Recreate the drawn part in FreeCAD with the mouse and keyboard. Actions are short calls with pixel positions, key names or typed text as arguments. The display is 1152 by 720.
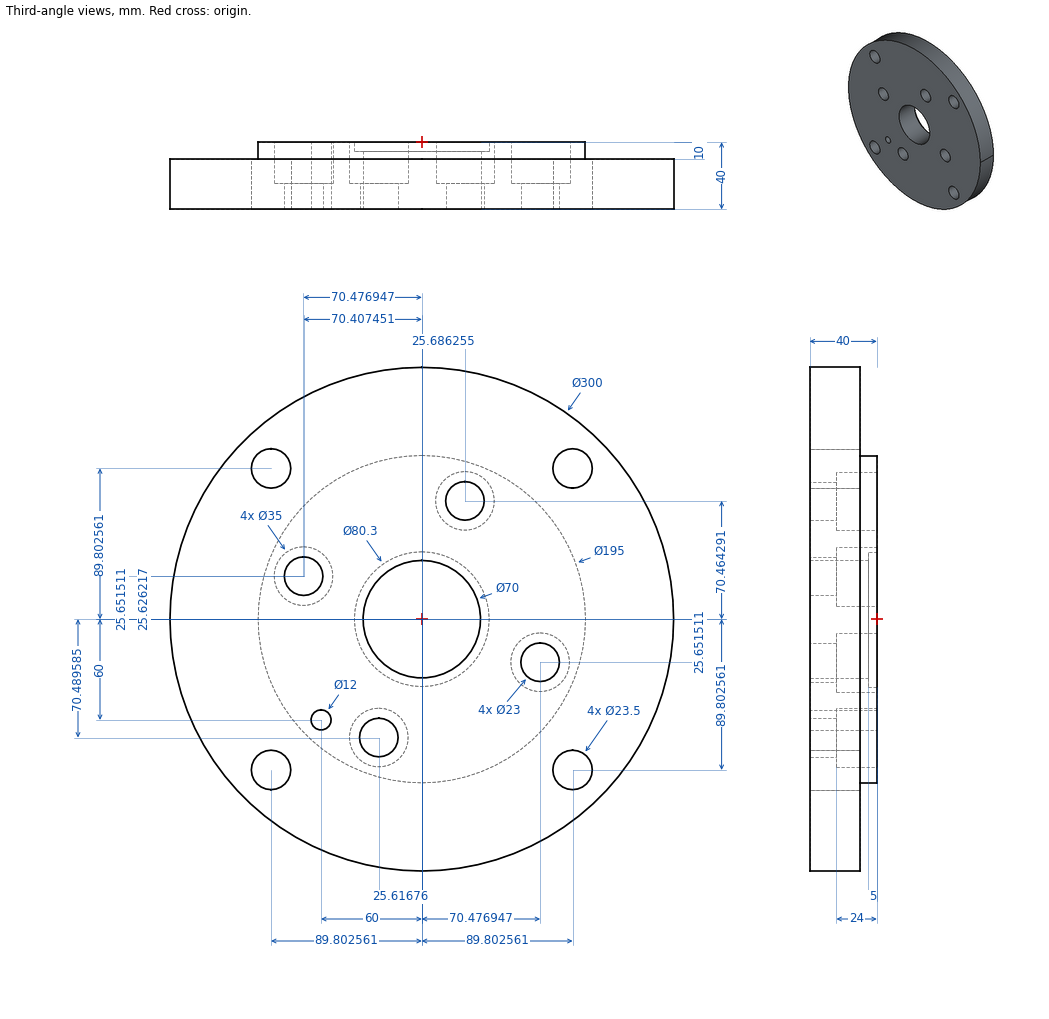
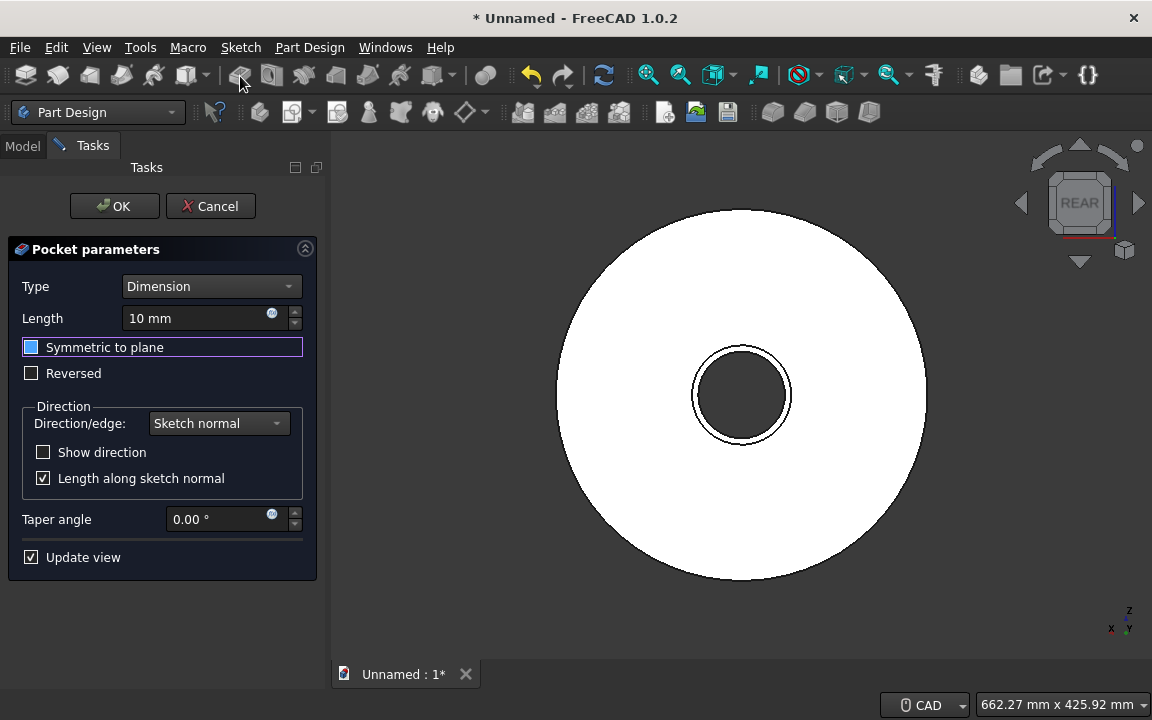
click(30, 373)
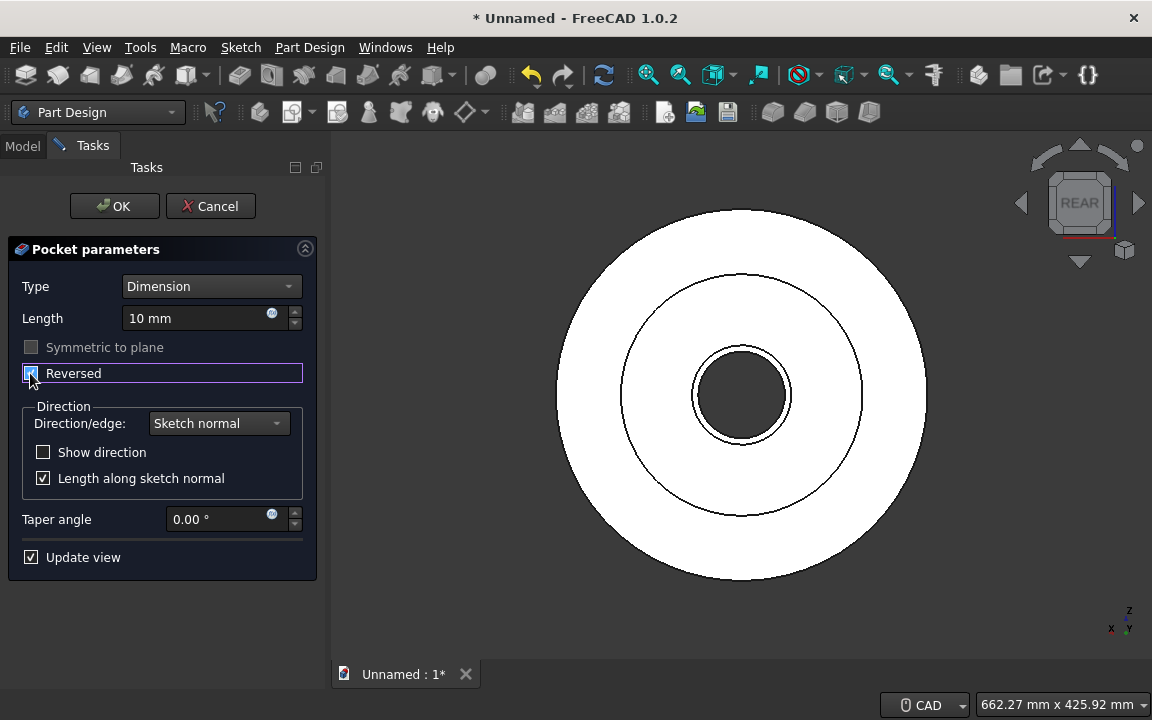
click(115, 206)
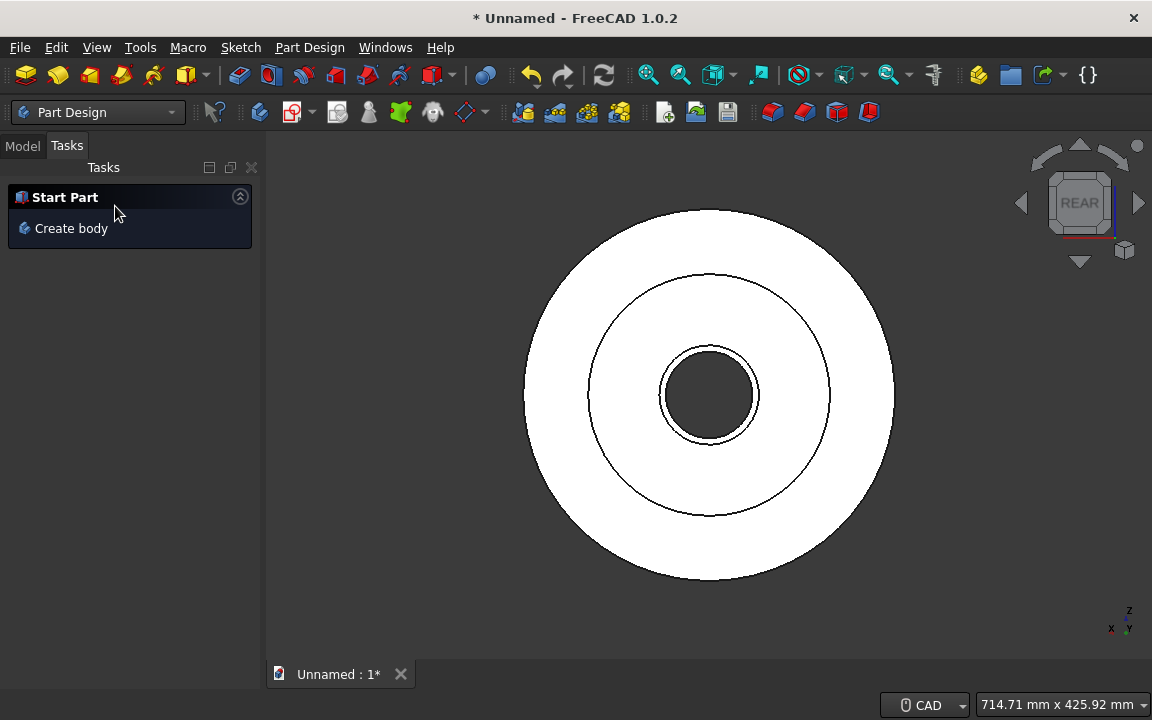
click(815, 288)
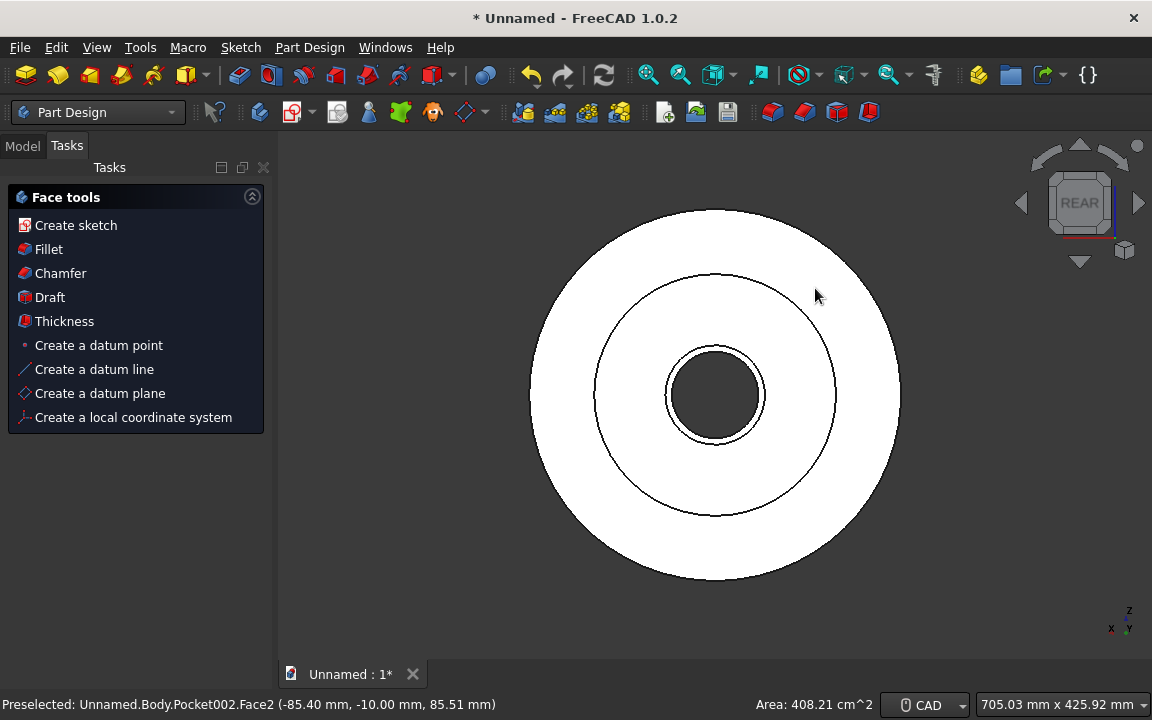
click(292, 112)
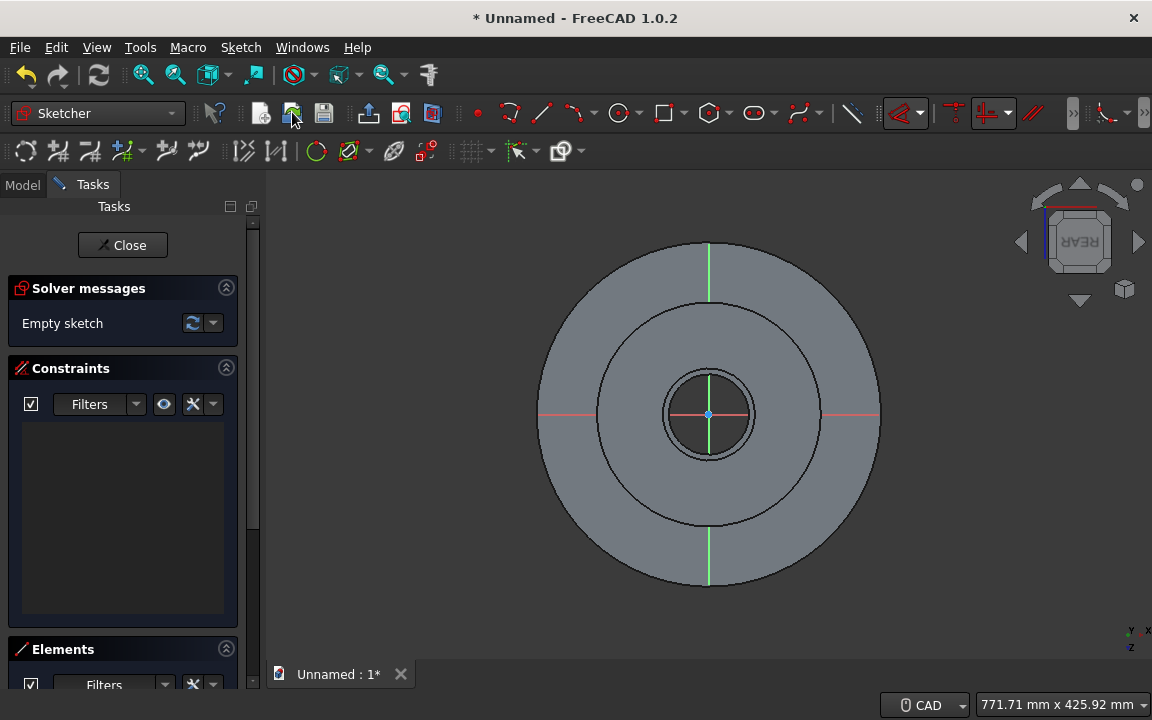
click(434, 114)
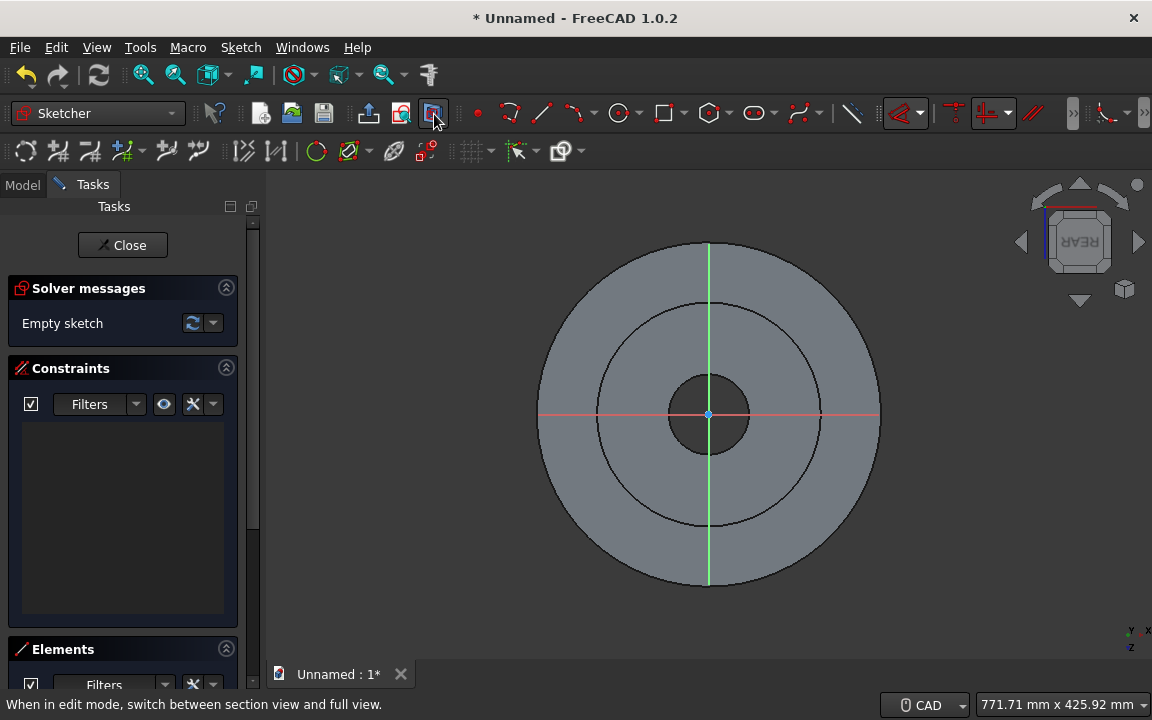
click(620, 114)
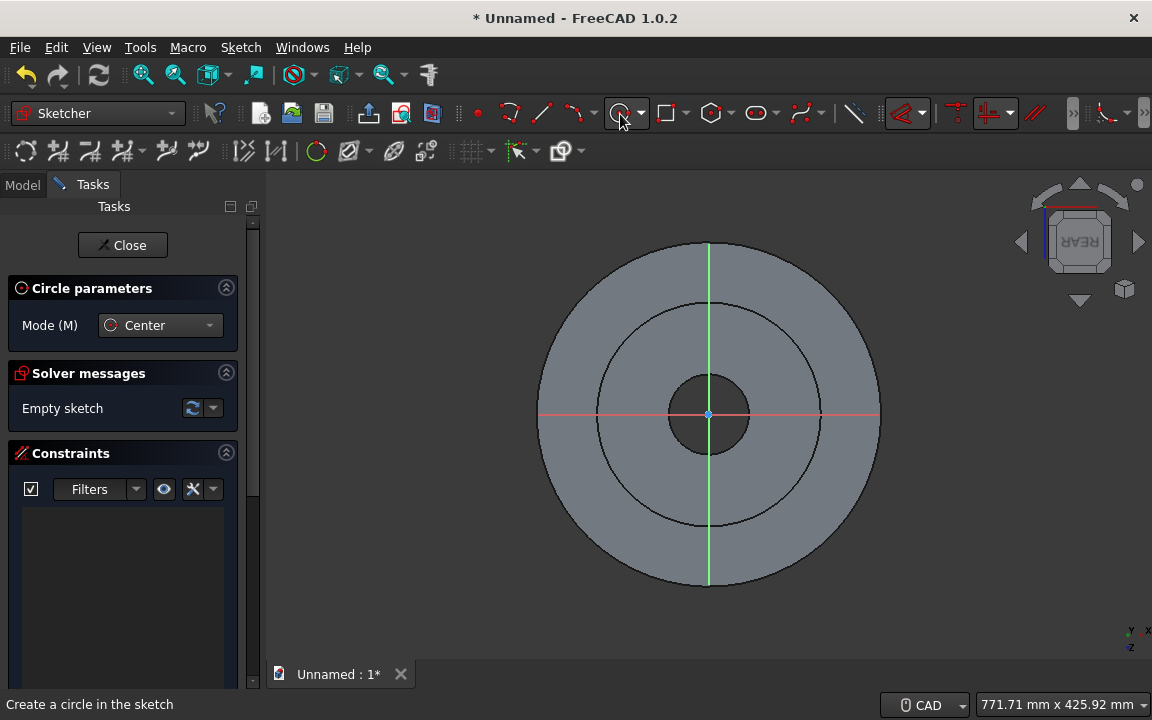
scroll(812, 311, up, 3)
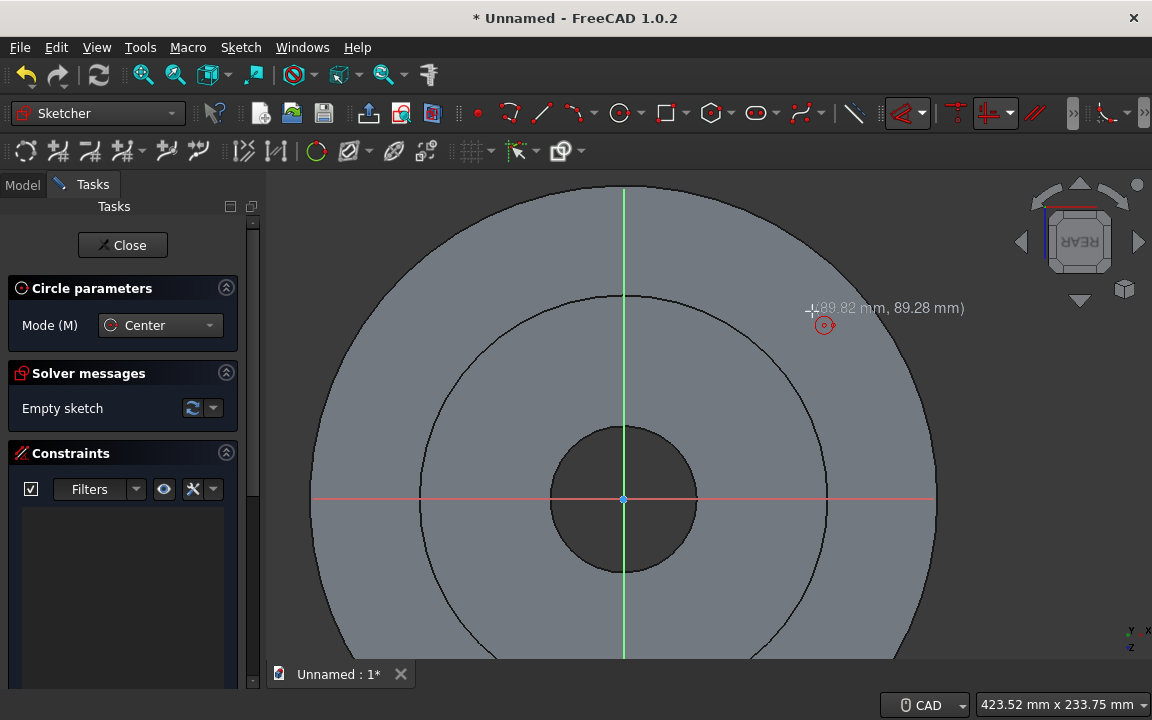
click(811, 311)
move(829, 294)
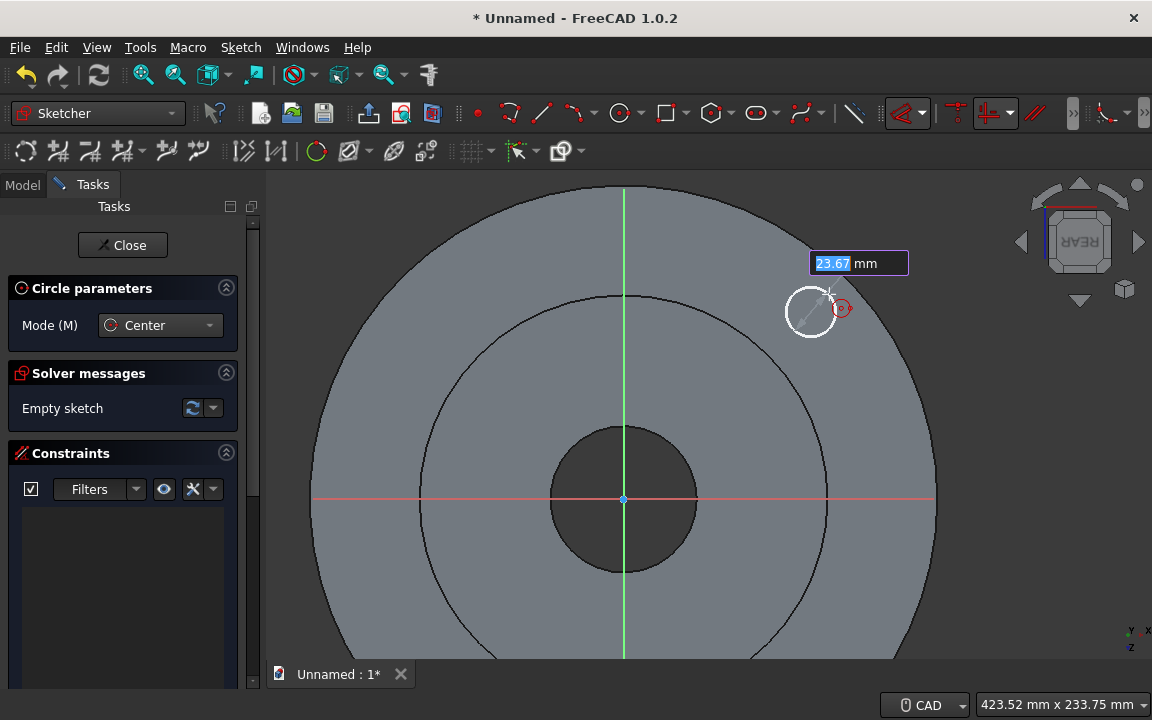
text(23.5)
key(Return)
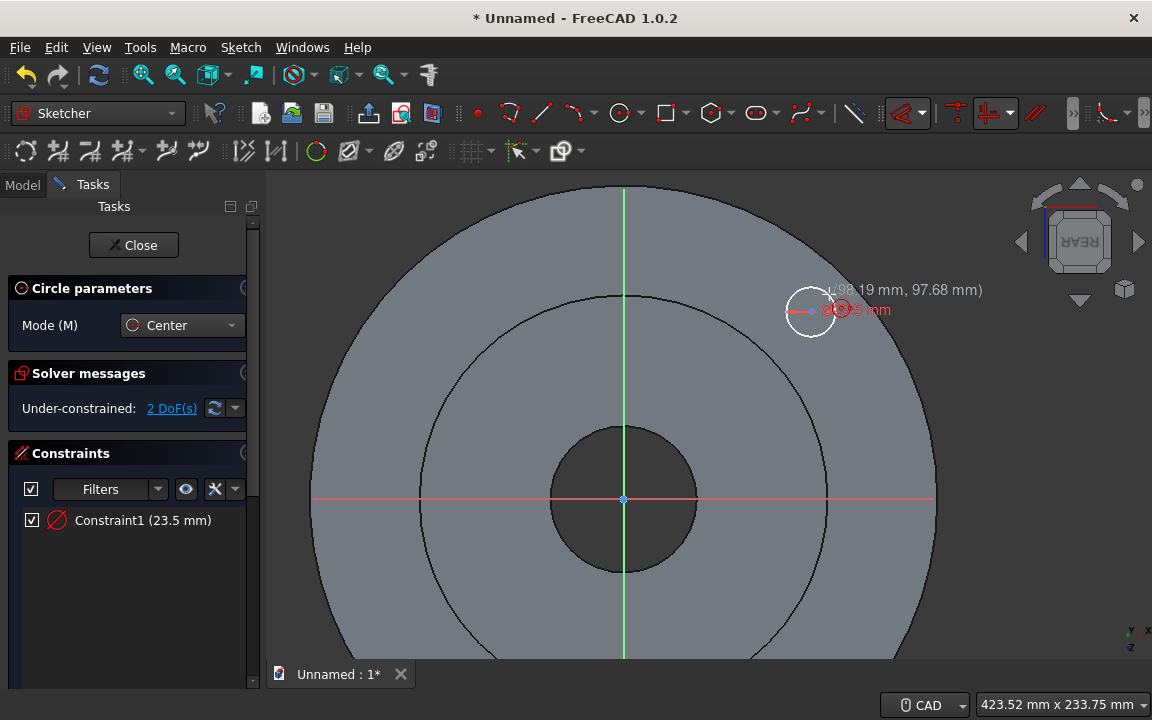
click(436, 311)
move(453, 294)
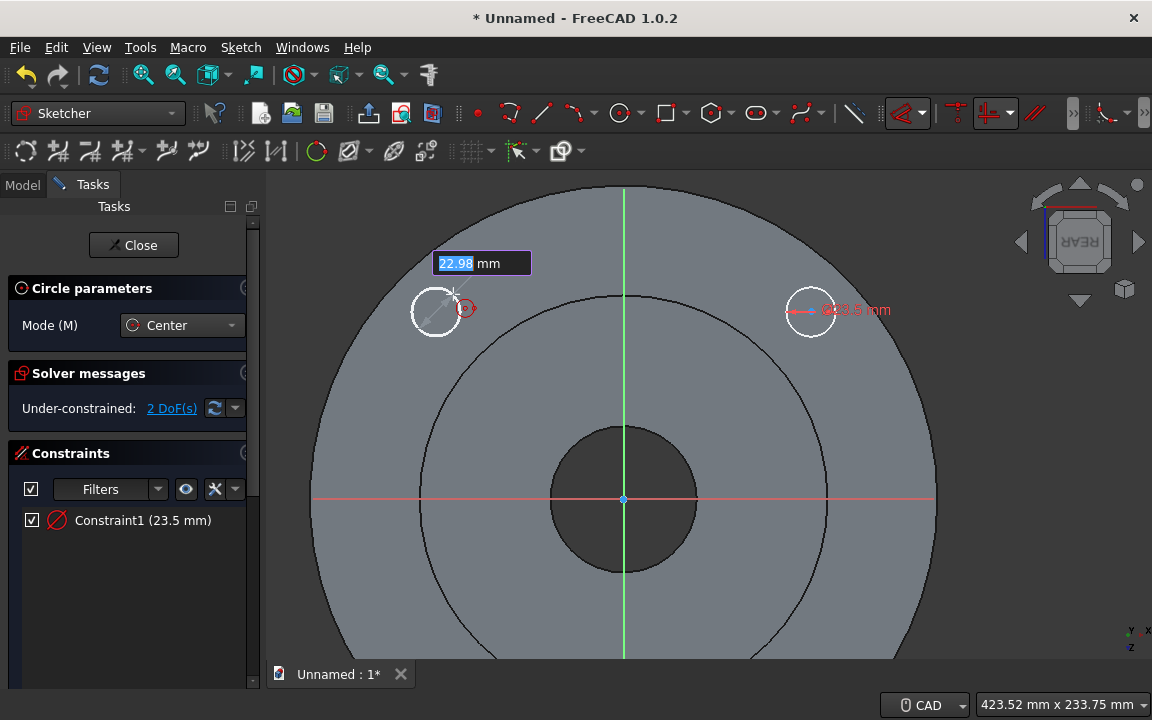
text(23.5)
key(Return)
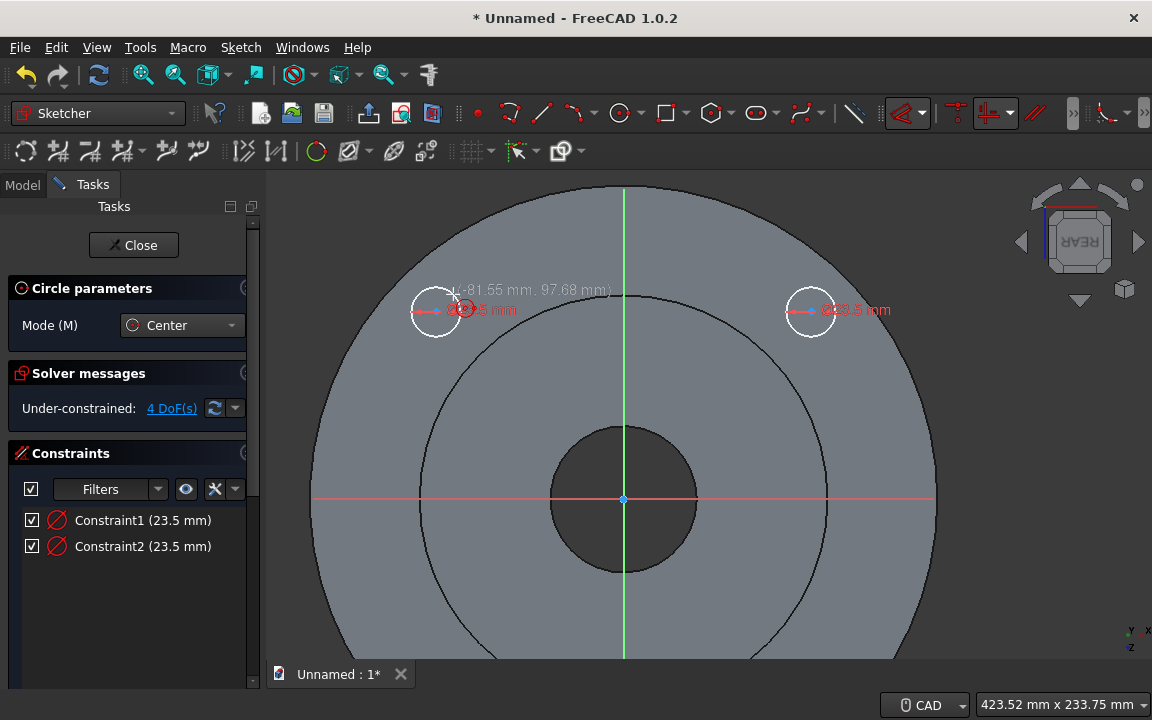
scroll(675, 242, down, 2)